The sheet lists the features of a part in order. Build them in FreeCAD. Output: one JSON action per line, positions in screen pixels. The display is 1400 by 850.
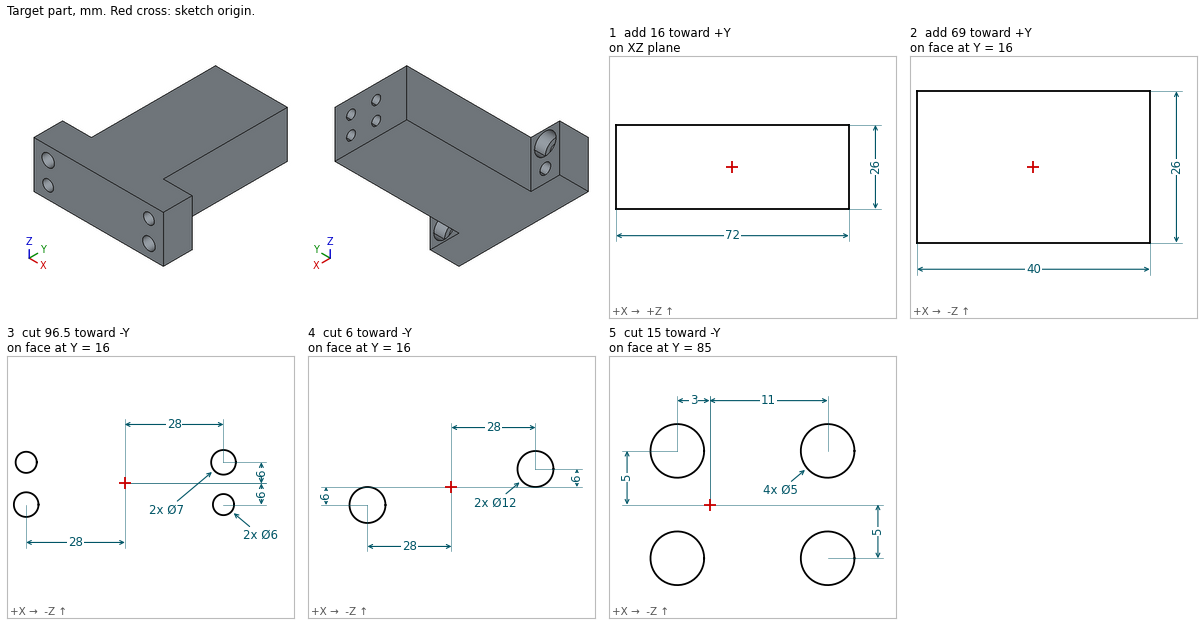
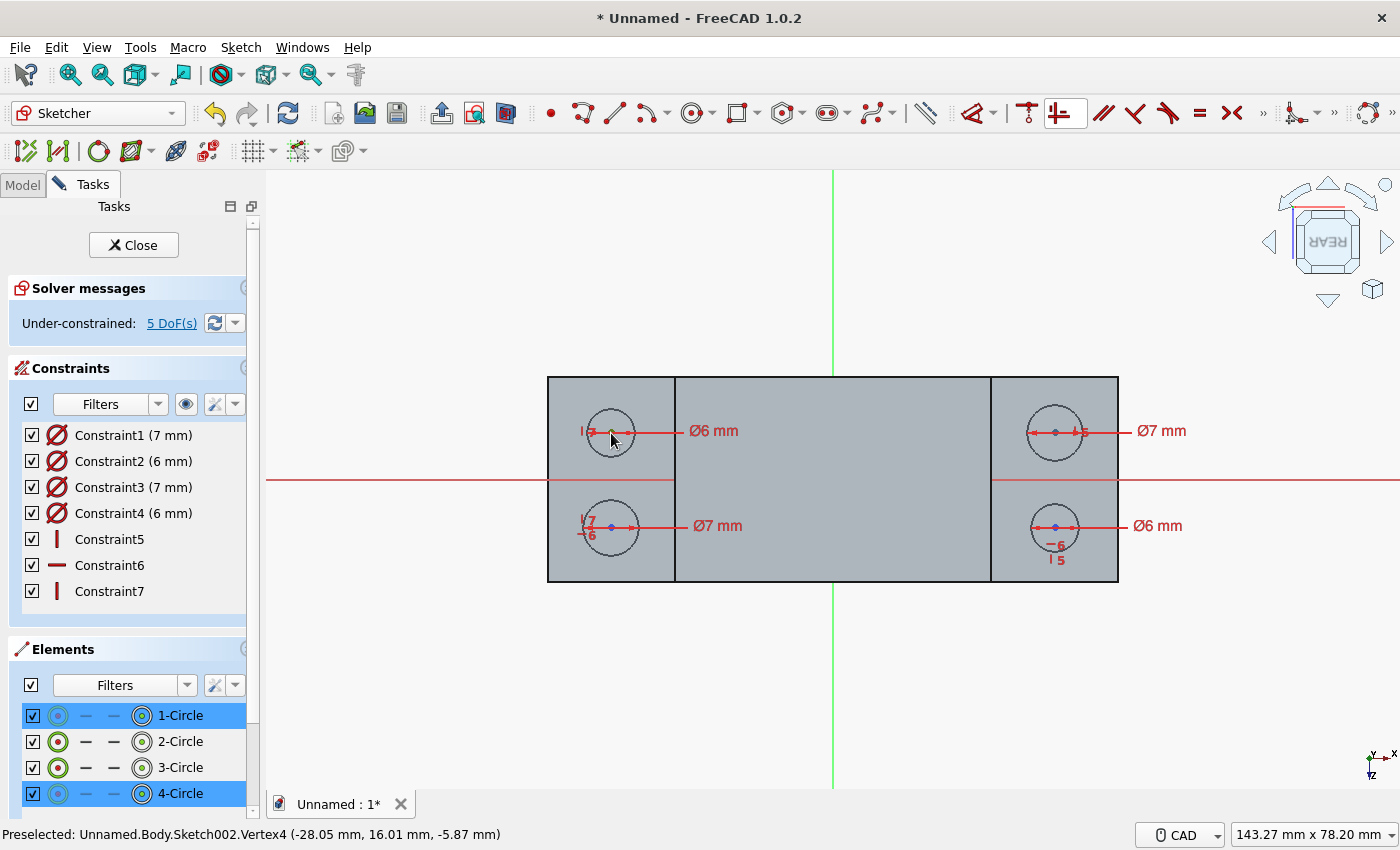
{"action": "left_click", "coordinate": [1082, 114]}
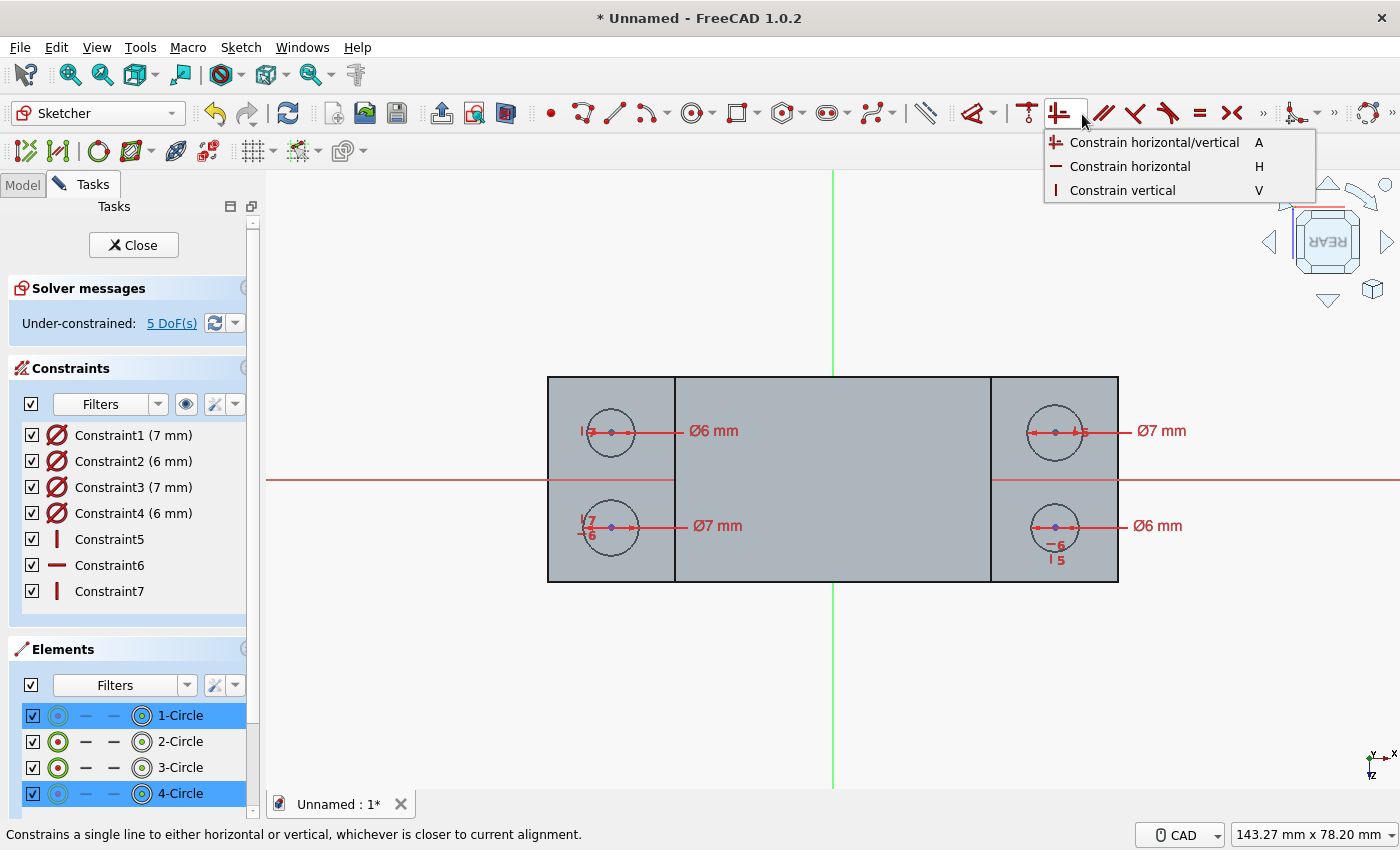
{"action": "left_click", "coordinate": [1180, 166]}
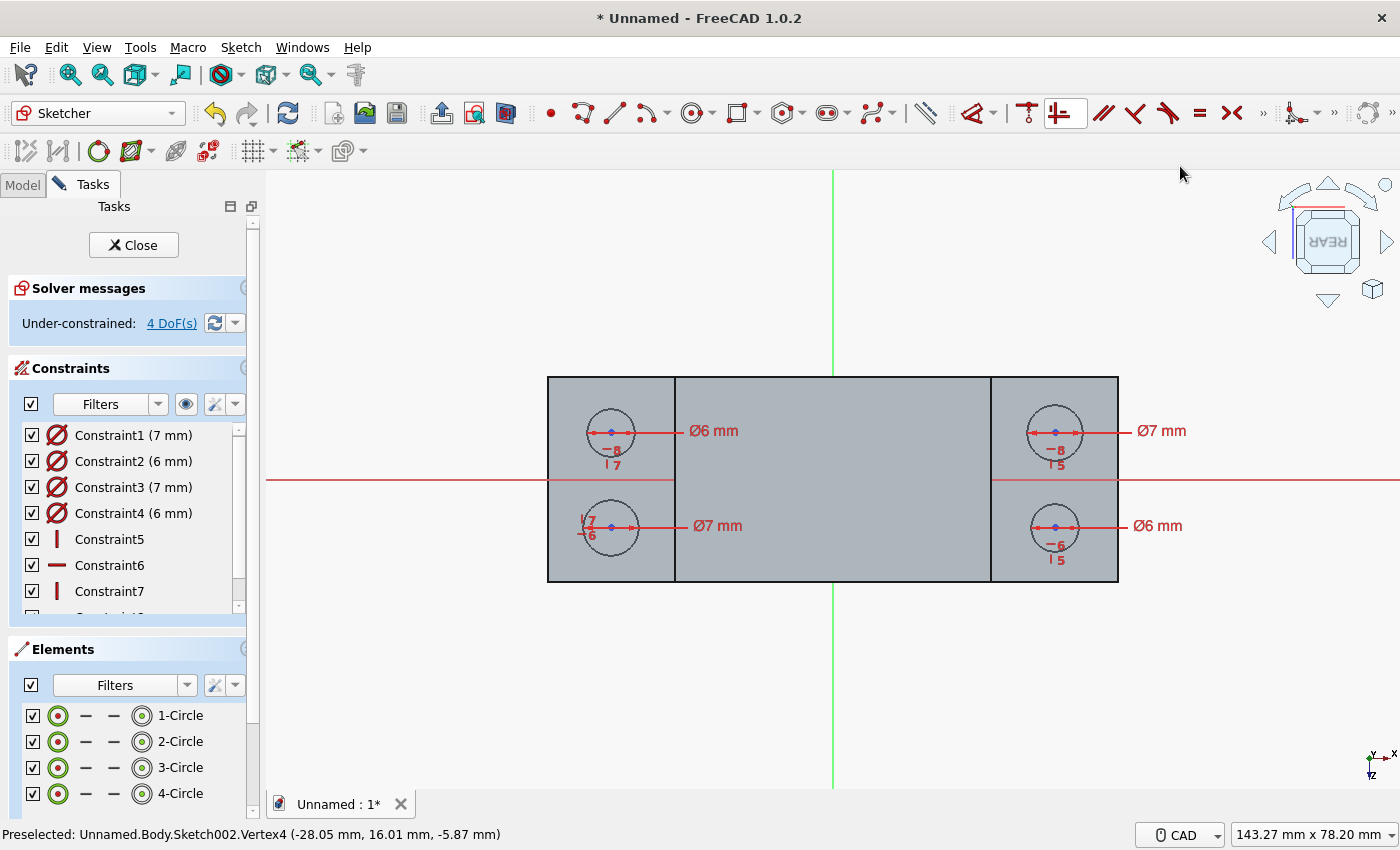
{"action": "left_click", "coordinate": [972, 114]}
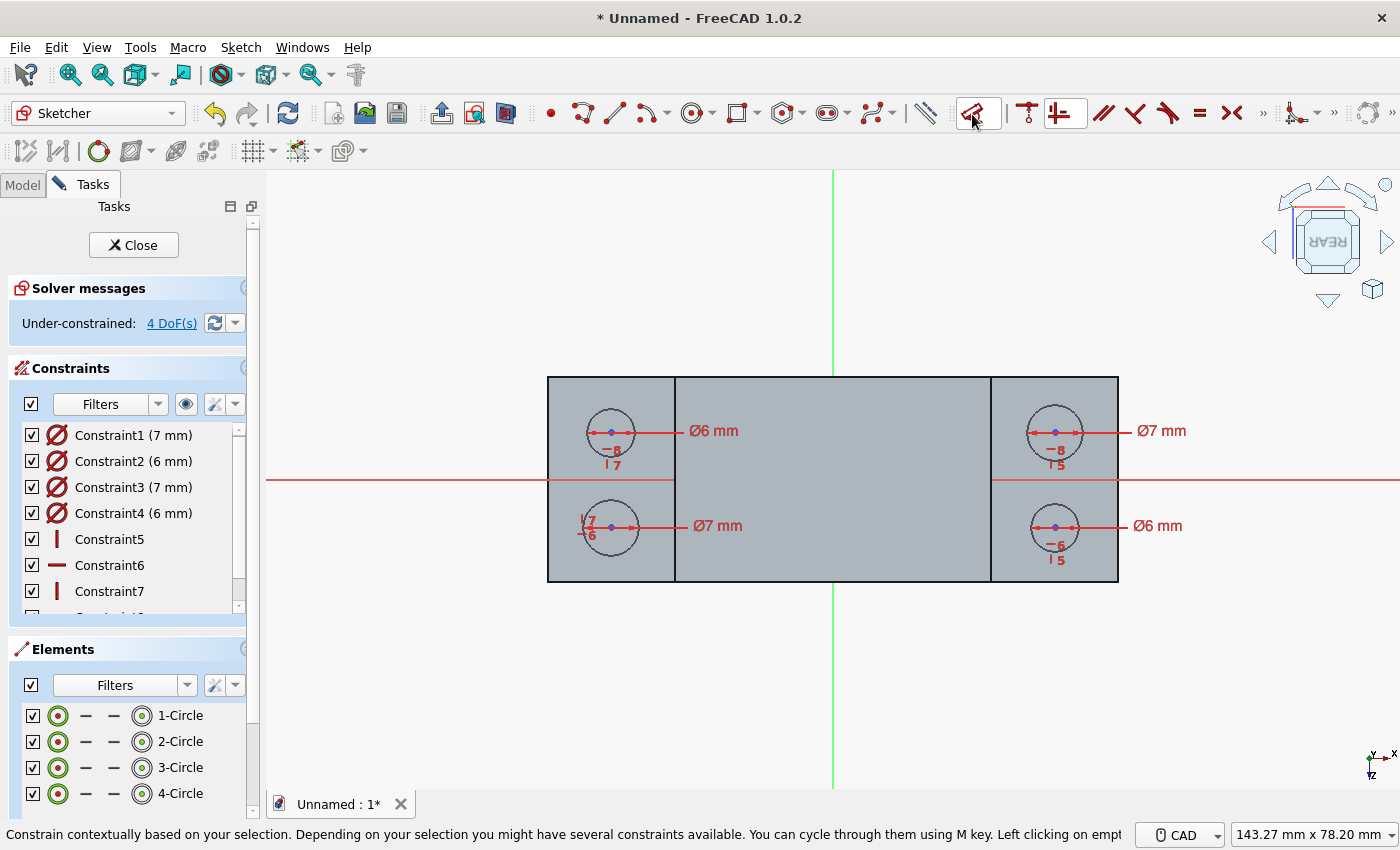
{"action": "left_click", "coordinate": [1055, 433]}
{"action": "left_click", "coordinate": [1089, 456]}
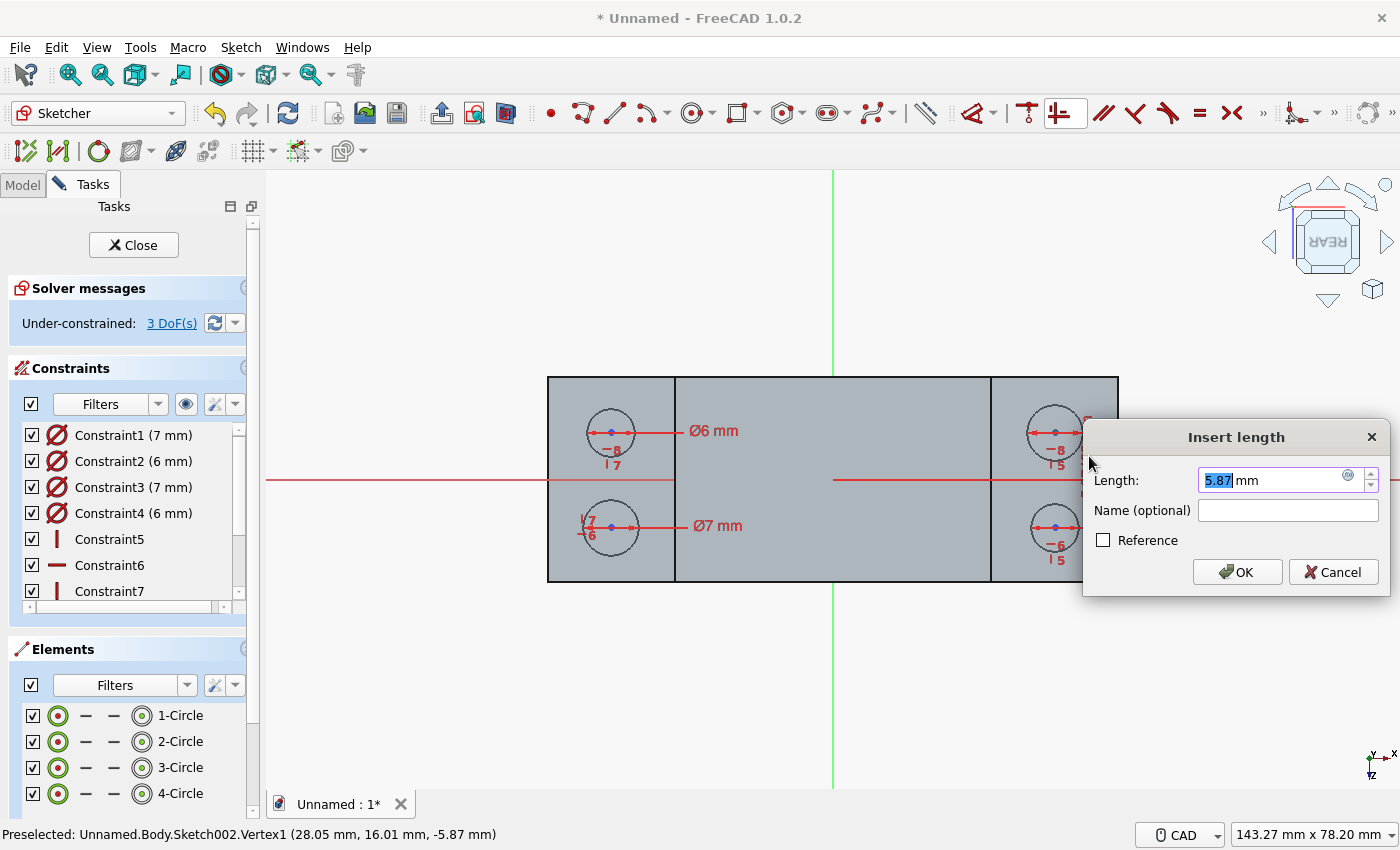
{"action": "type", "text": "6"}
{"action": "key", "text": "Return"}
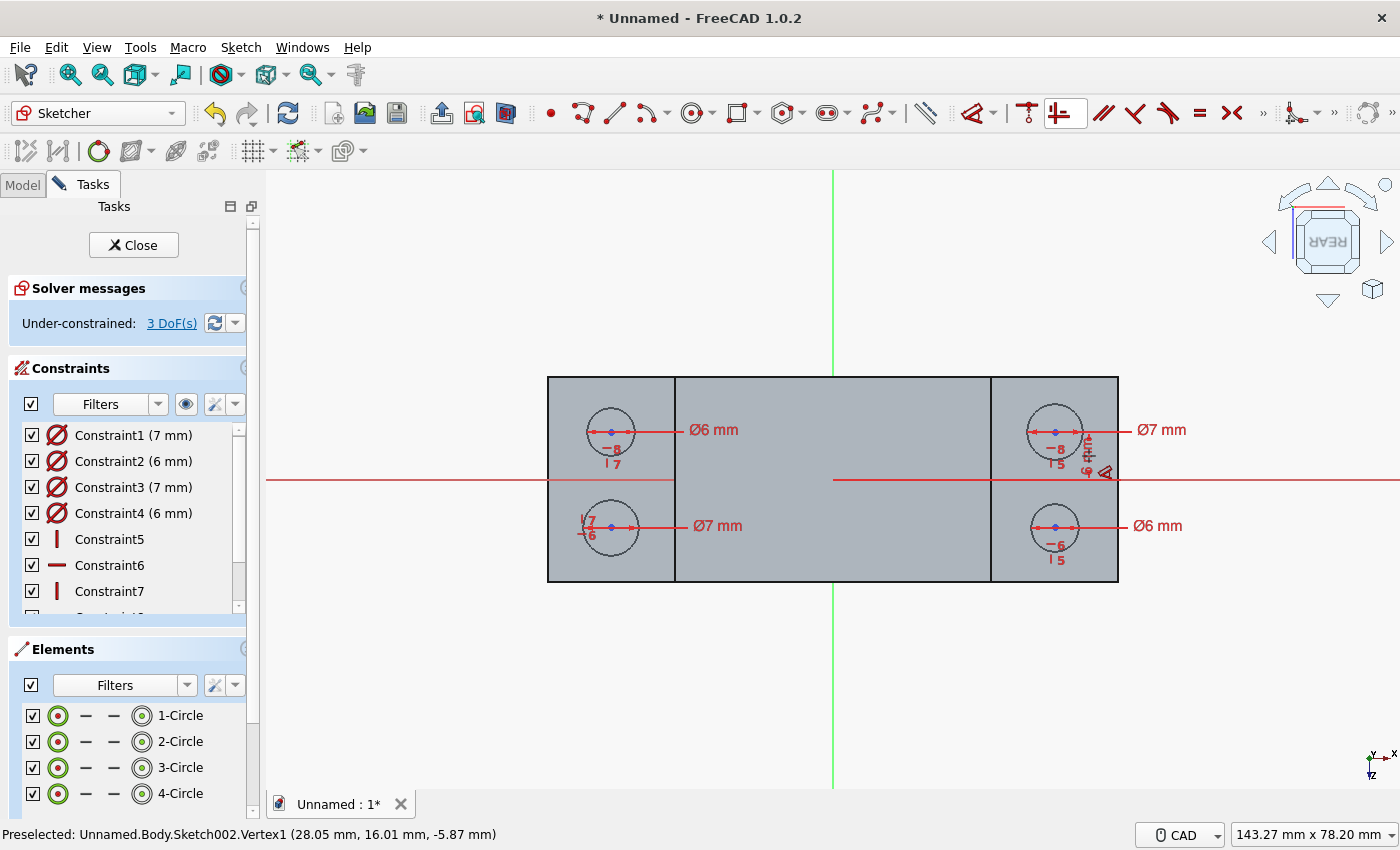
{"action": "left_click", "coordinate": [1055, 528]}
{"action": "left_click", "coordinate": [1089, 504]}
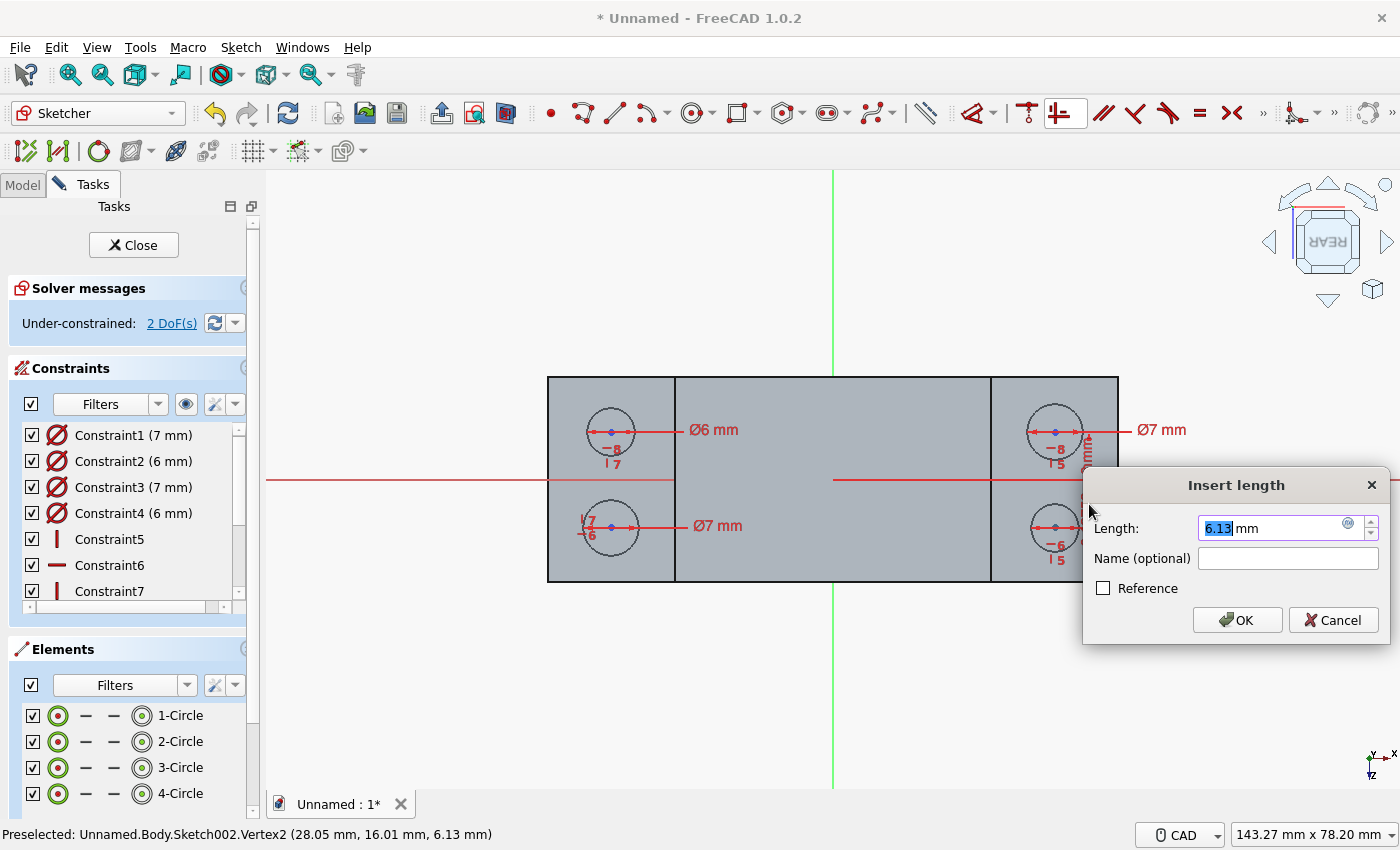
{"action": "type", "text": "6"}
{"action": "key", "text": "Return"}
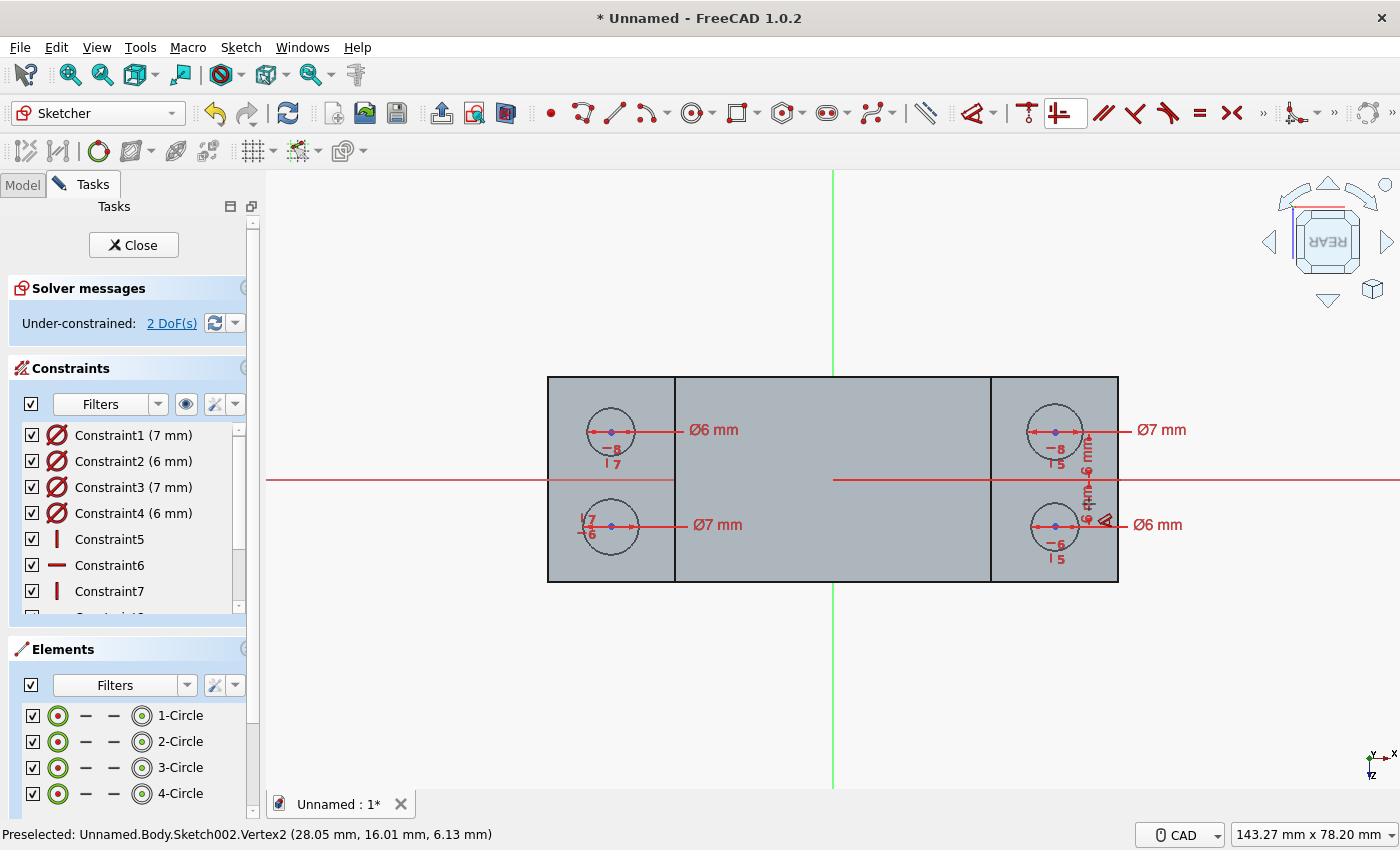
{"action": "left_click", "coordinate": [1055, 432]}
{"action": "left_click", "coordinate": [944, 398]}